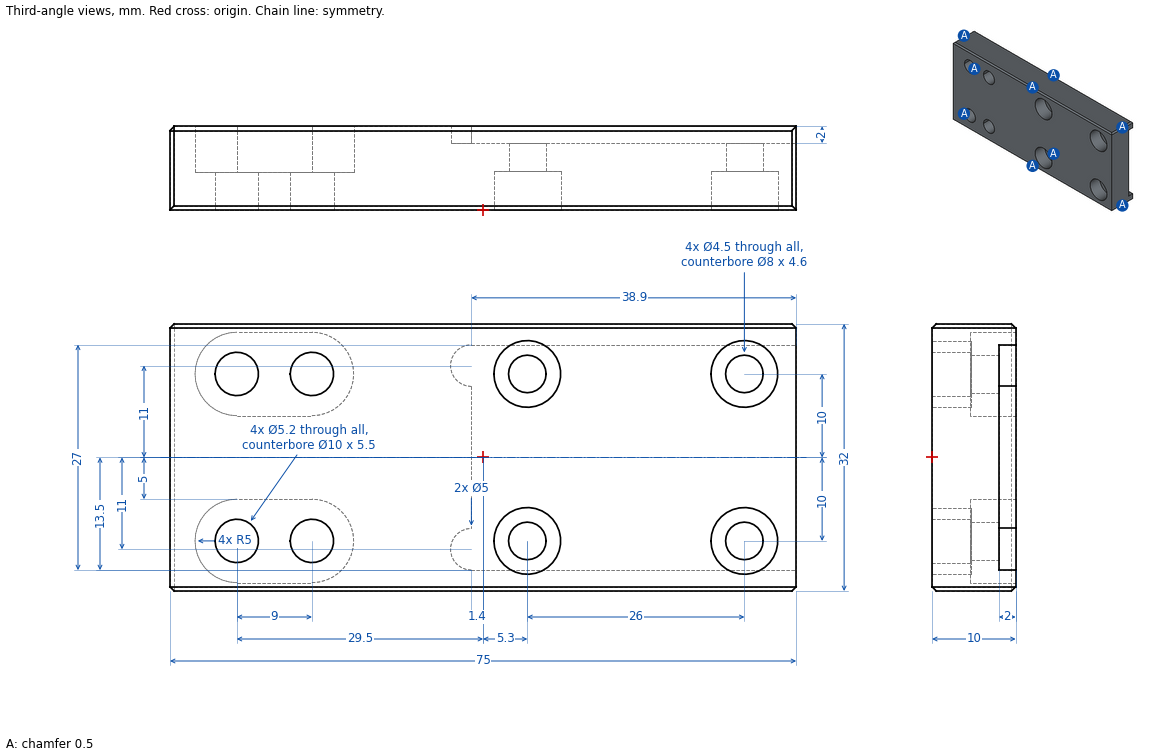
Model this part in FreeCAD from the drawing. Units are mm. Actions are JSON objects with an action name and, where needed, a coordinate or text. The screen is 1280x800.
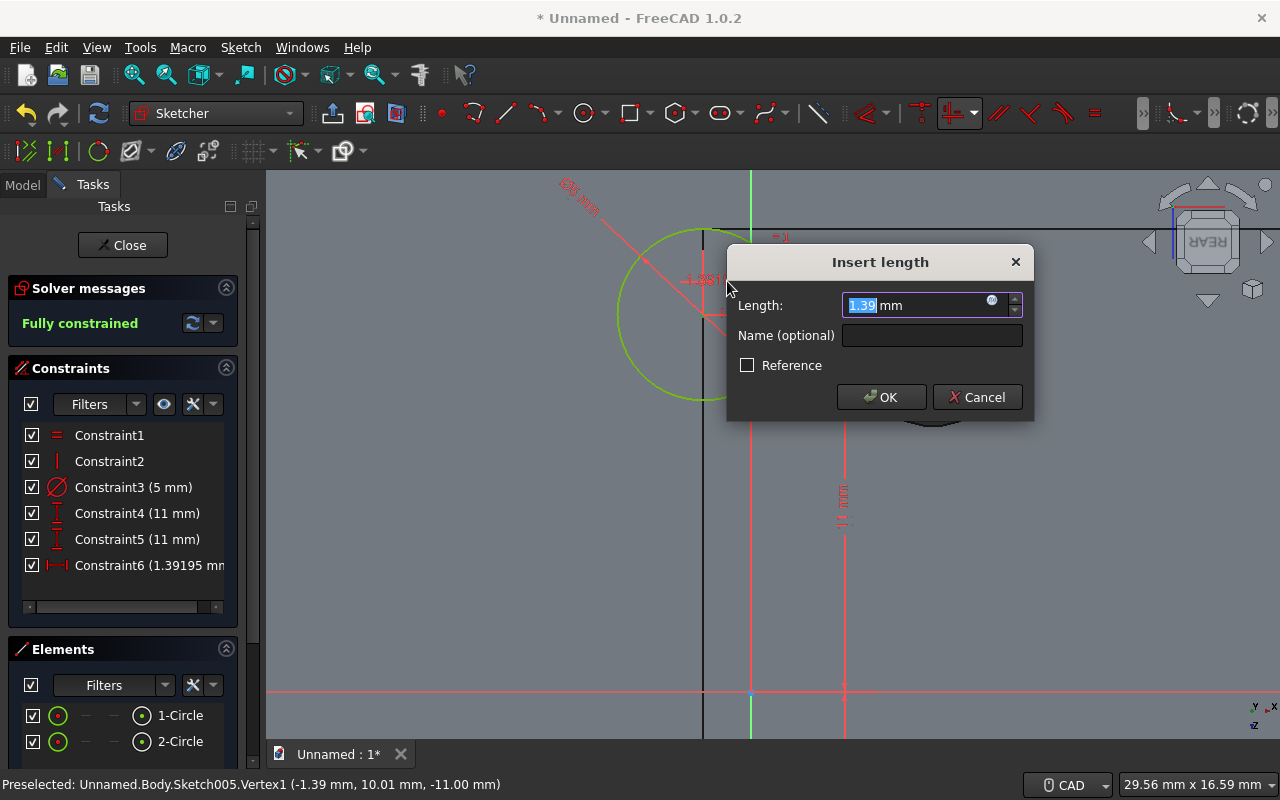
{"action": "type", "text": "1.4"}
{"action": "key", "text": "Return"}
{"action": "key", "text": "Escape"}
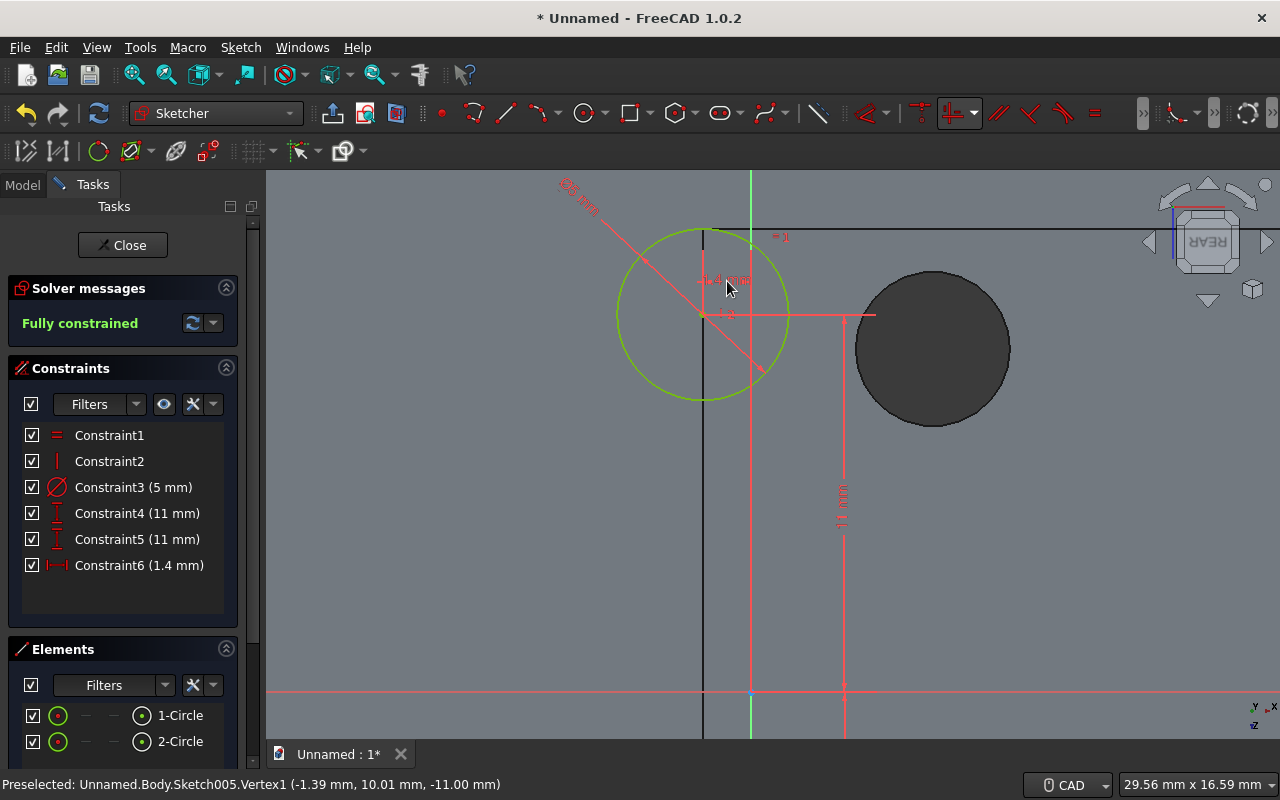
{"action": "left_click", "coordinate": [123, 245]}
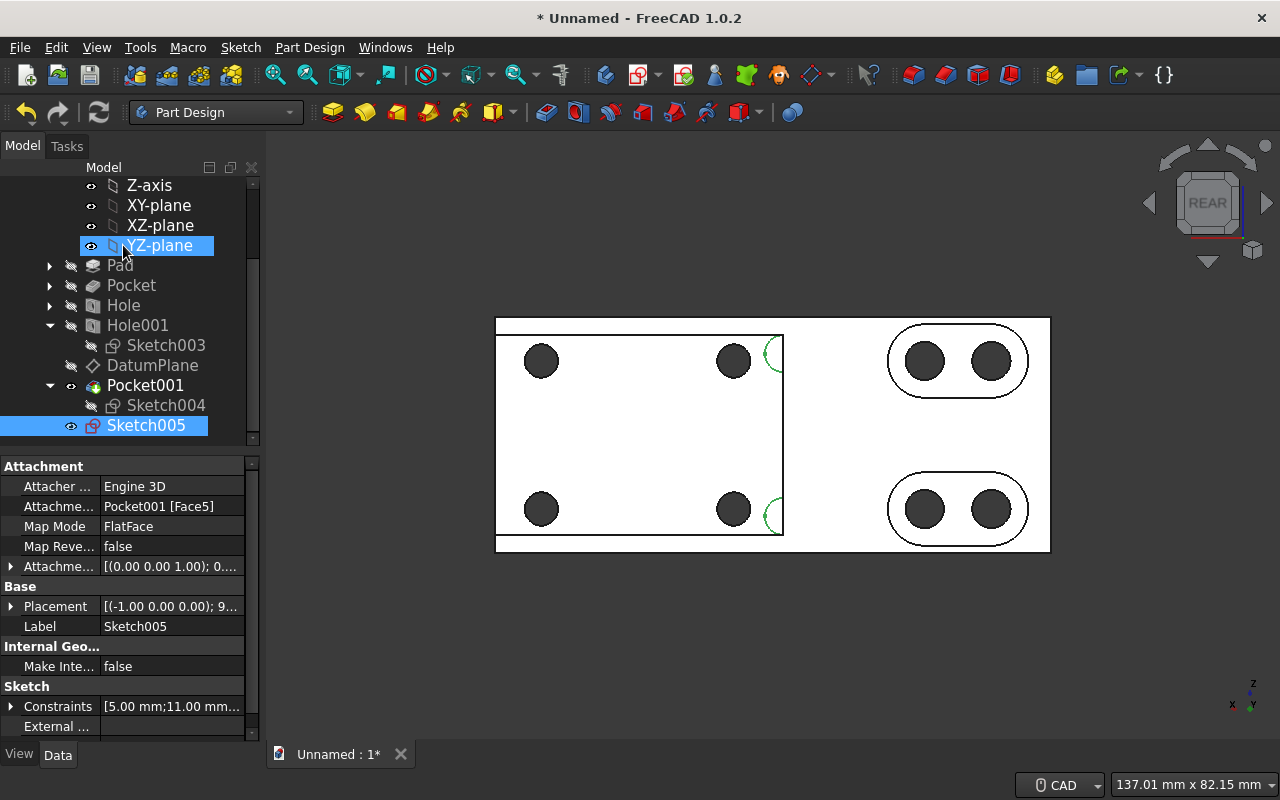
{"action": "left_click", "coordinate": [548, 112]}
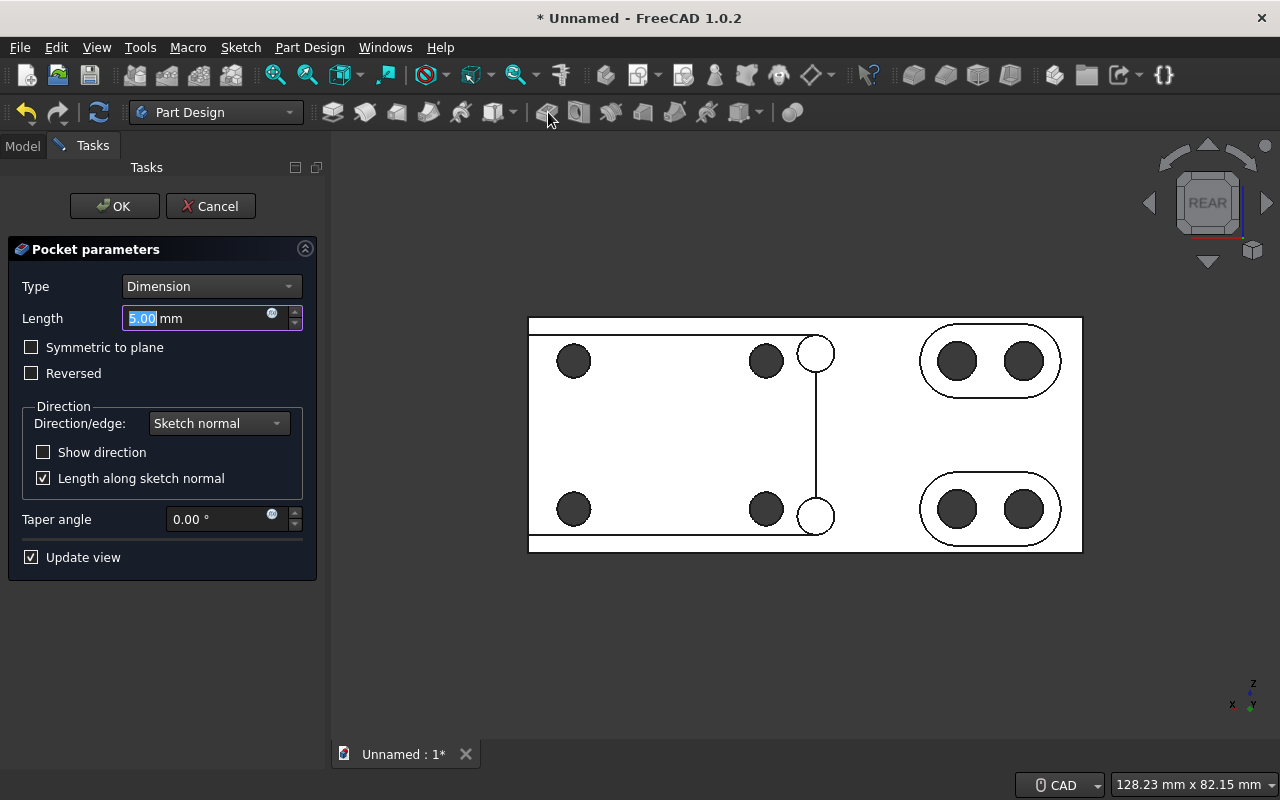
{"action": "type", "text": "2"}
{"action": "key", "text": "Tab"}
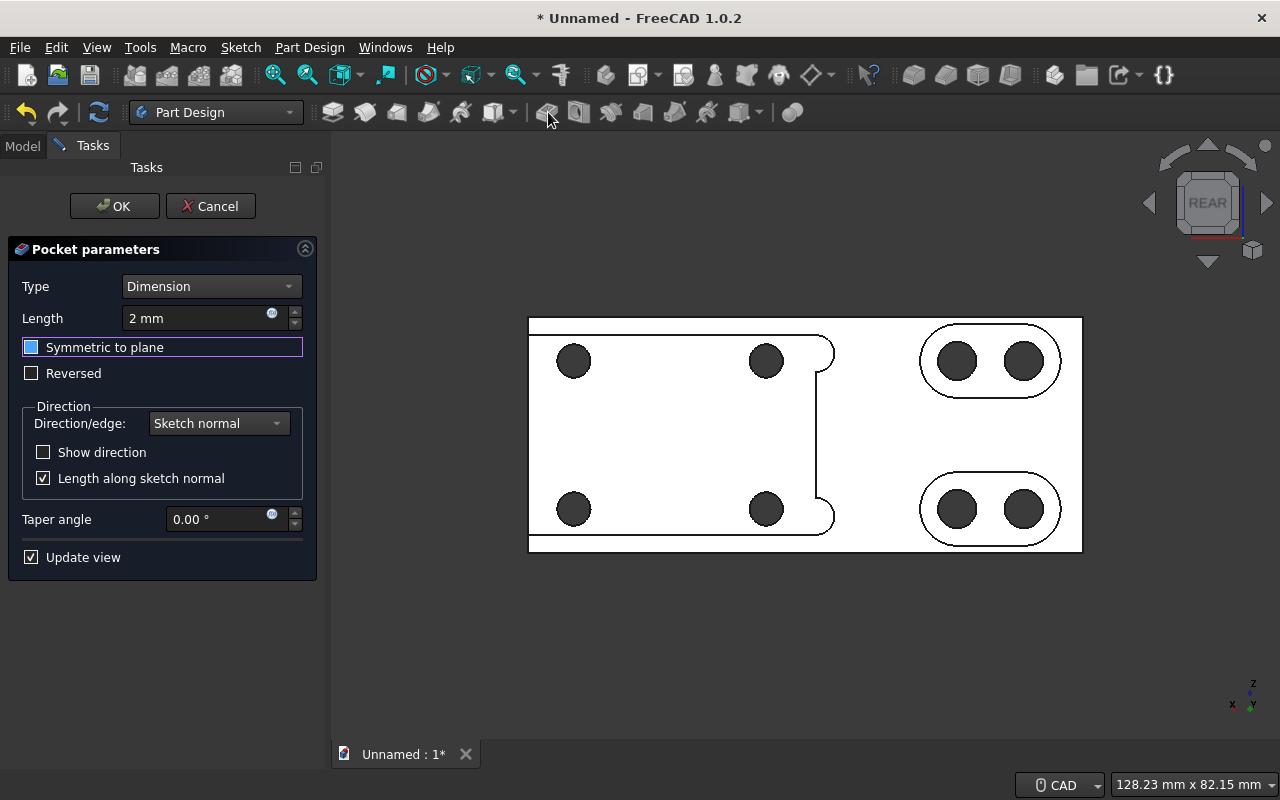
{"action": "left_click", "coordinate": [115, 206]}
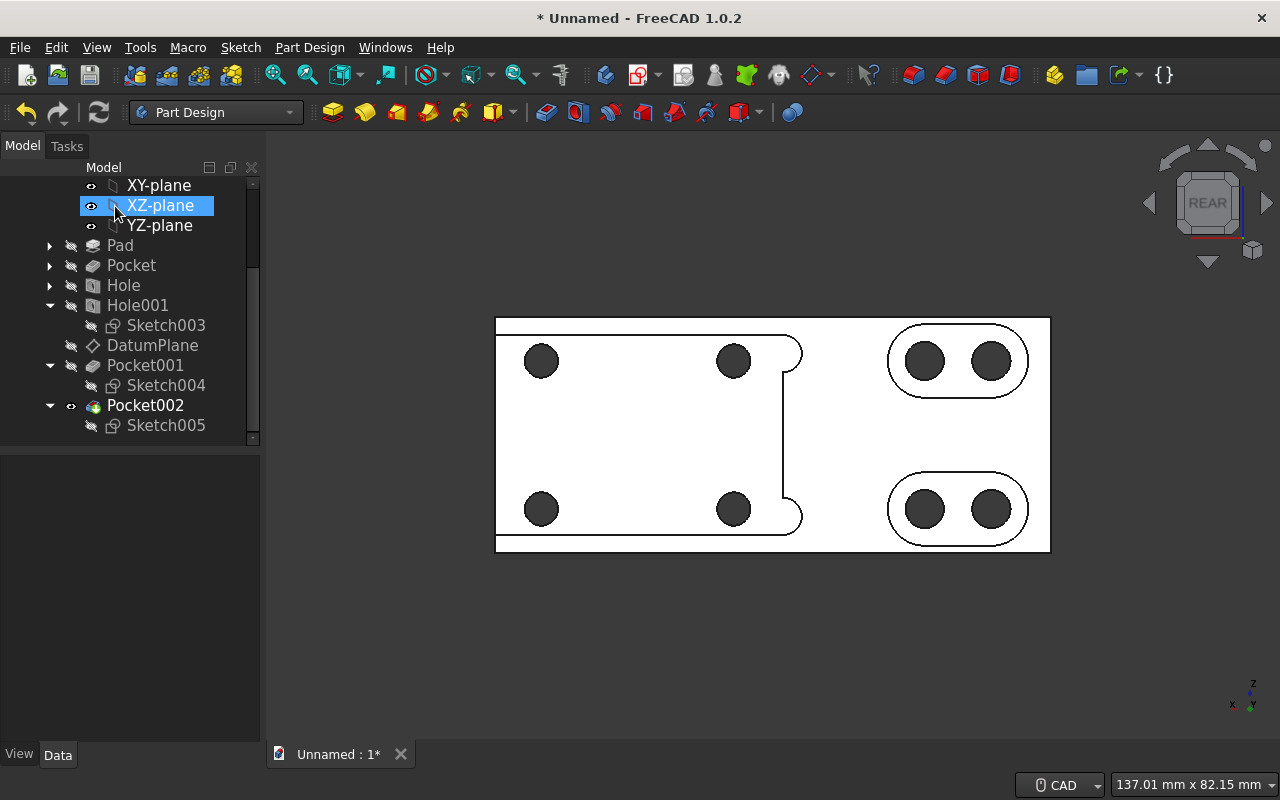
{"action": "left_click", "coordinate": [1051, 434]}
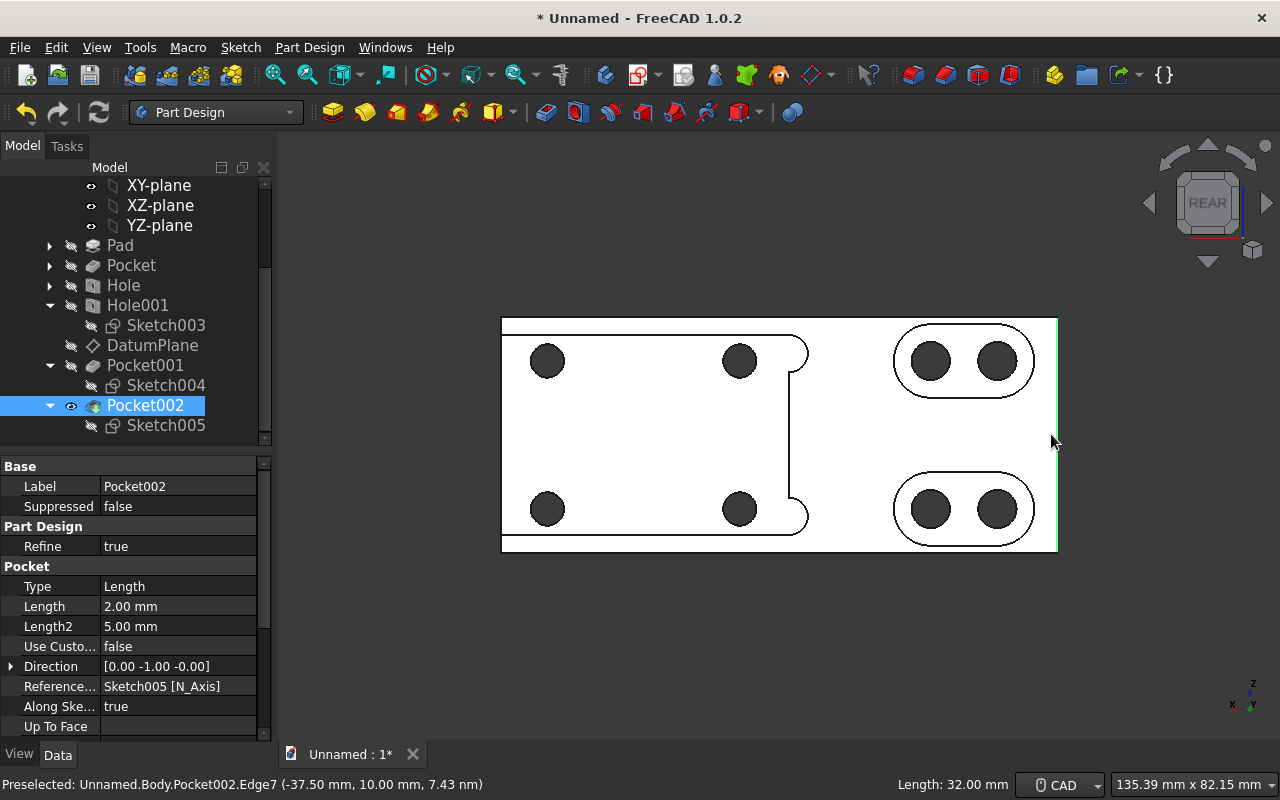
{"action": "key", "text": "0"}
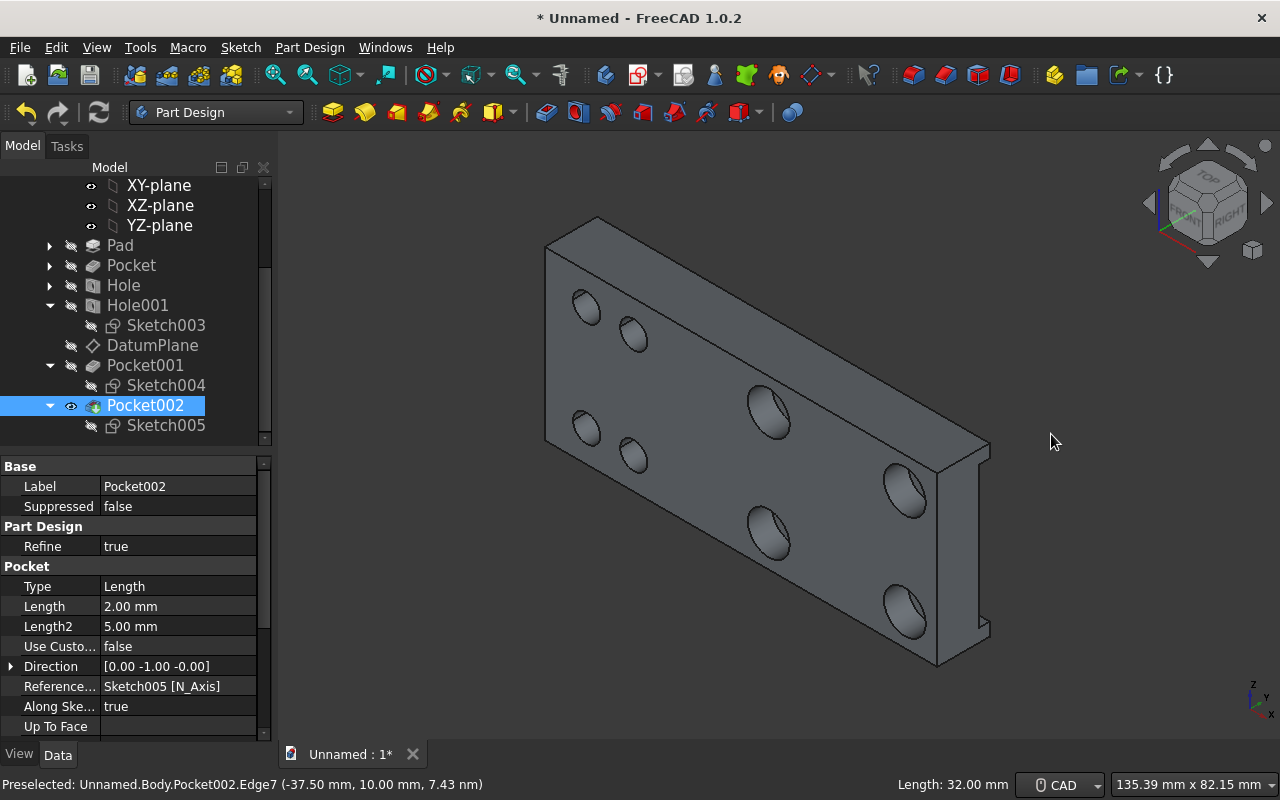
{"action": "left_click", "coordinate": [935, 441], "text": "ctrl"}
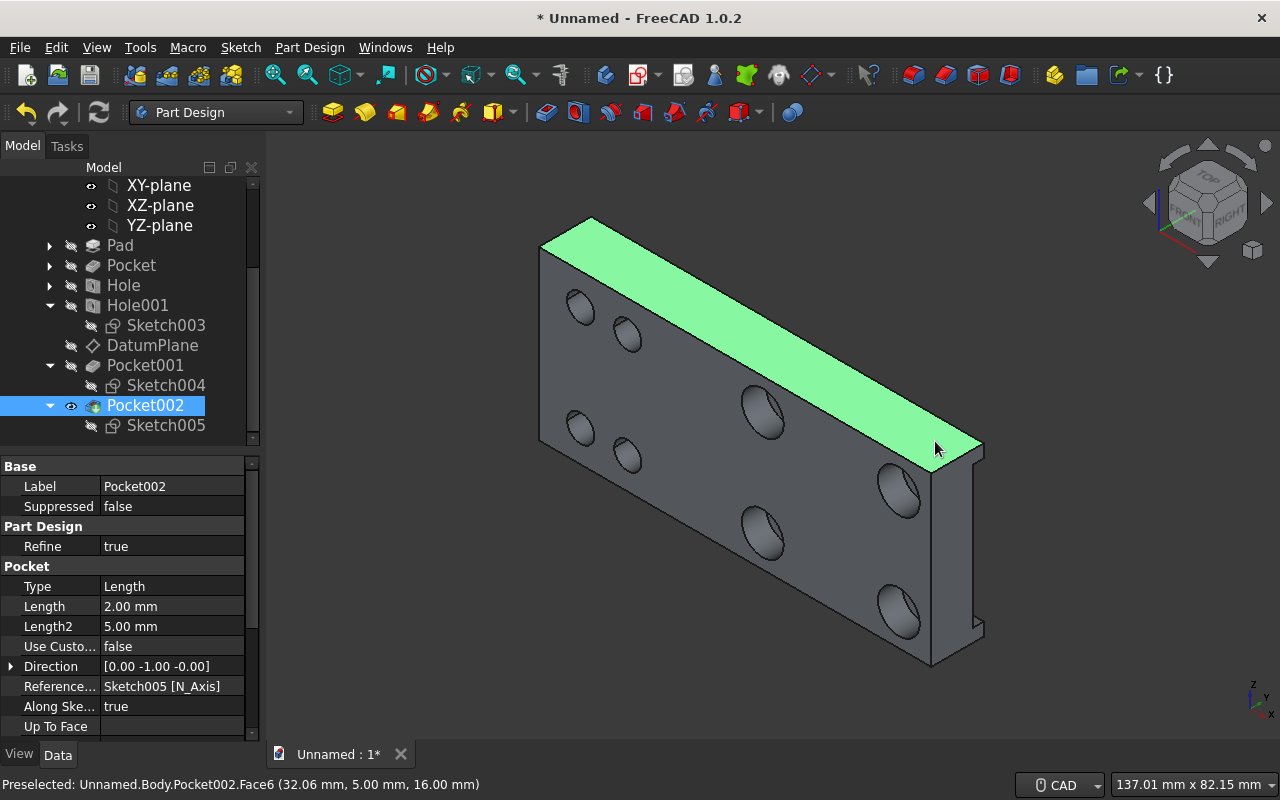
{"action": "key", "text": "2"}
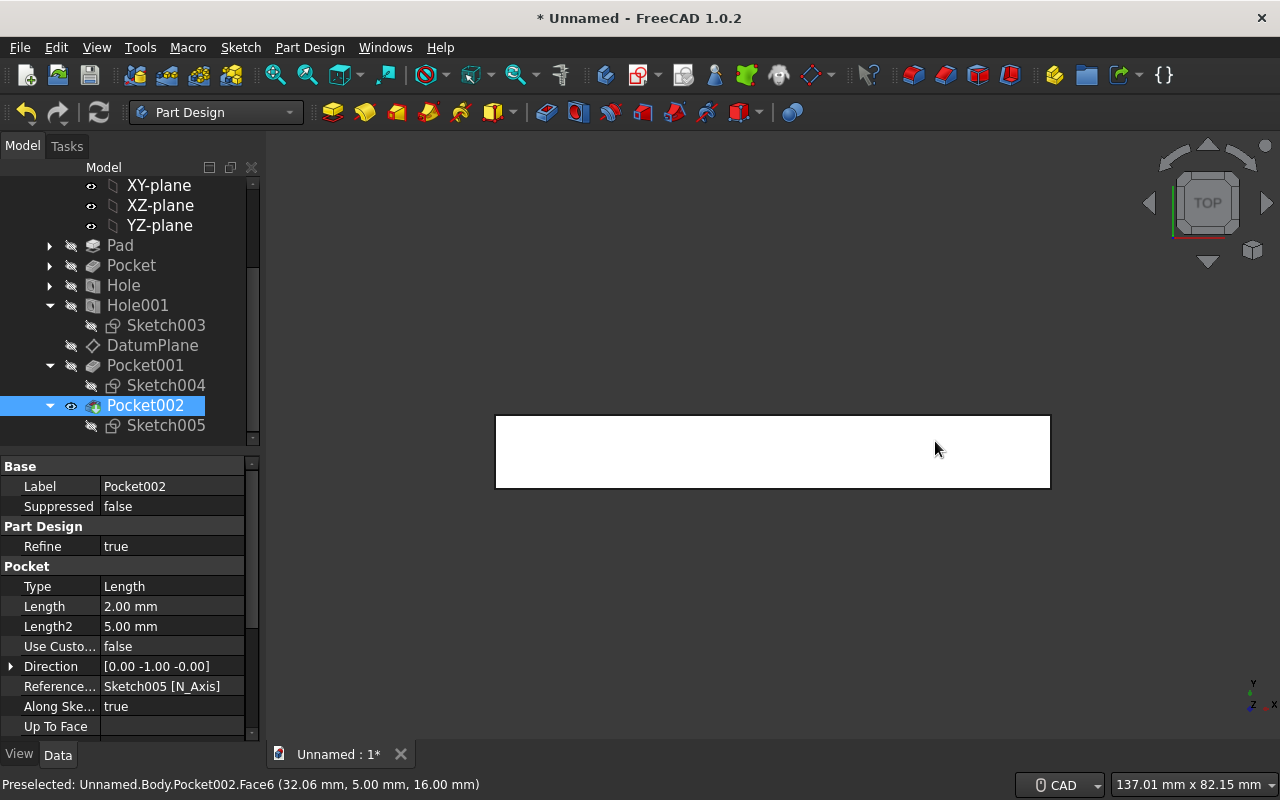
{"action": "key", "text": "1"}